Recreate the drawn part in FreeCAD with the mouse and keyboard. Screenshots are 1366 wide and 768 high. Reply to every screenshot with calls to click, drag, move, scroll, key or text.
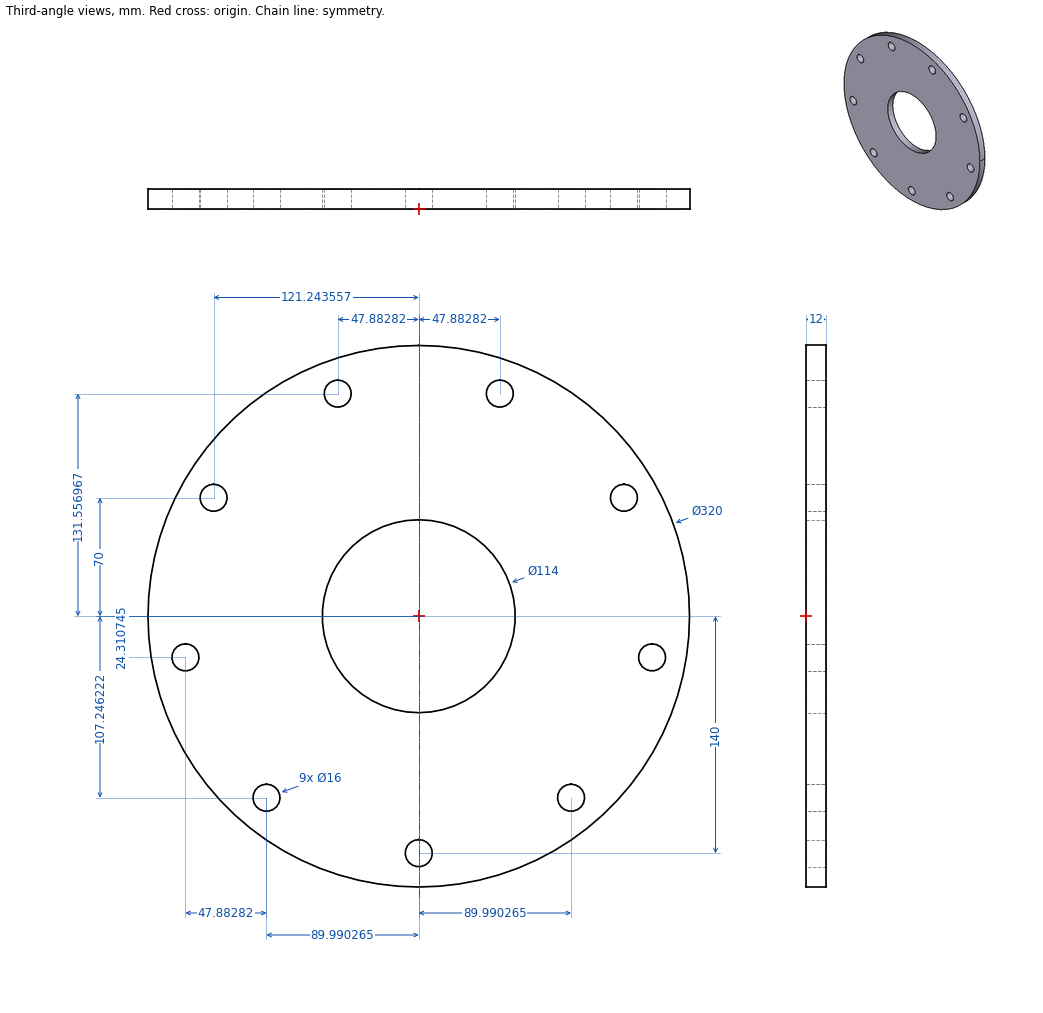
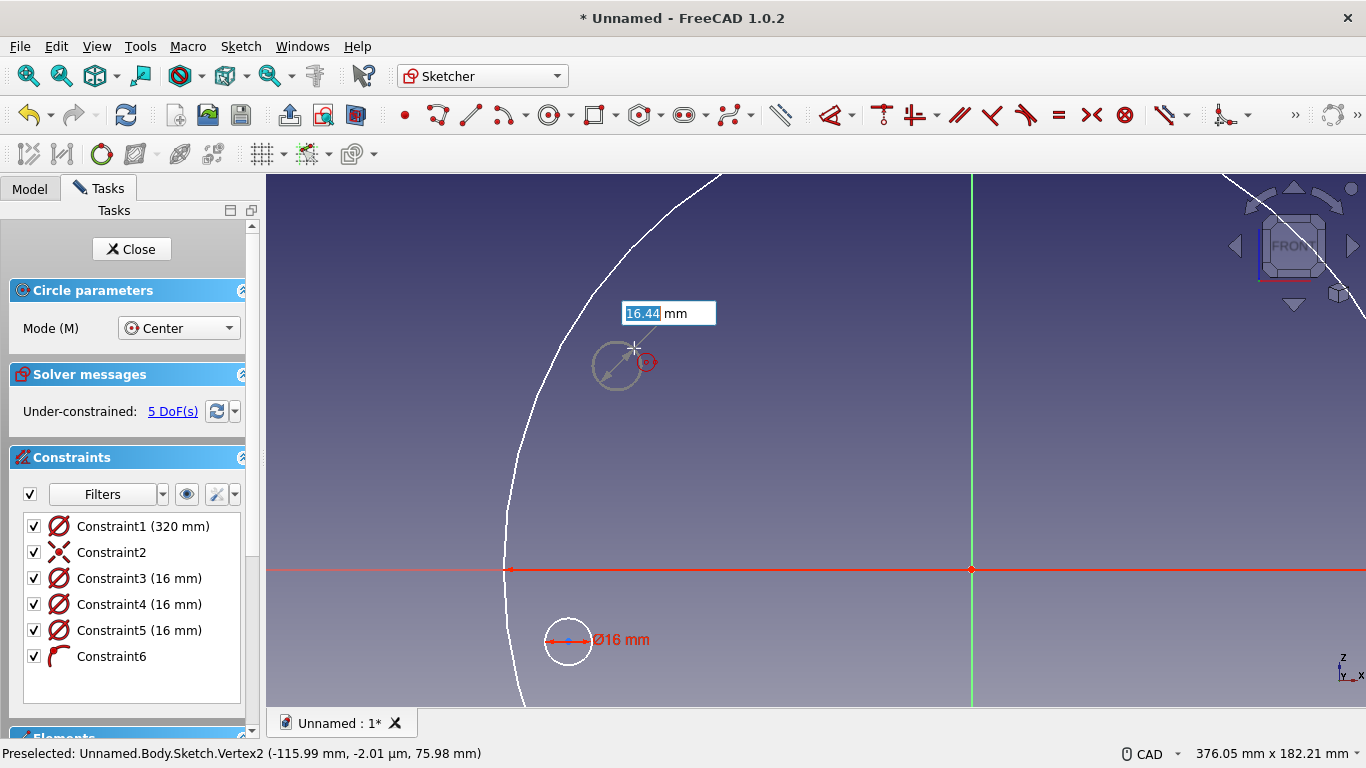
text(16)
key(Return)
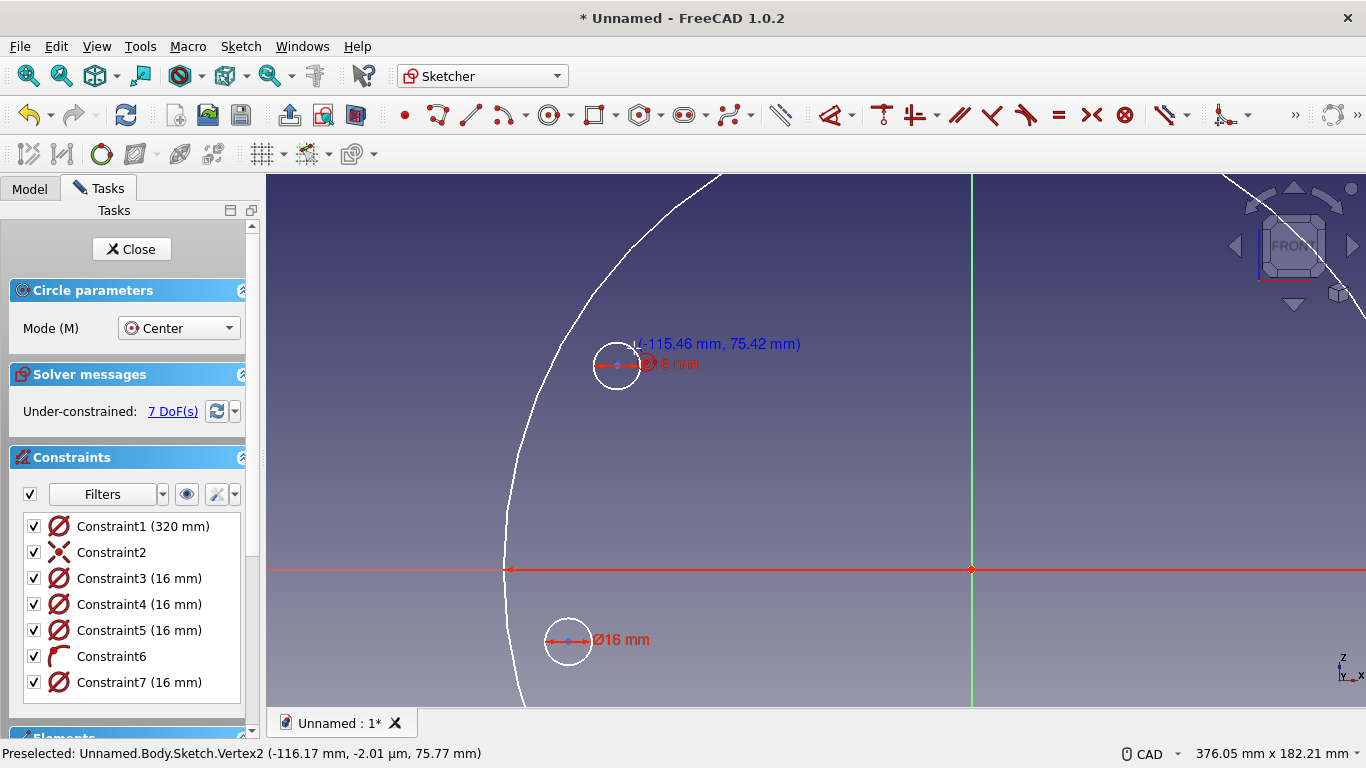
click(972, 570)
move(1090, 452)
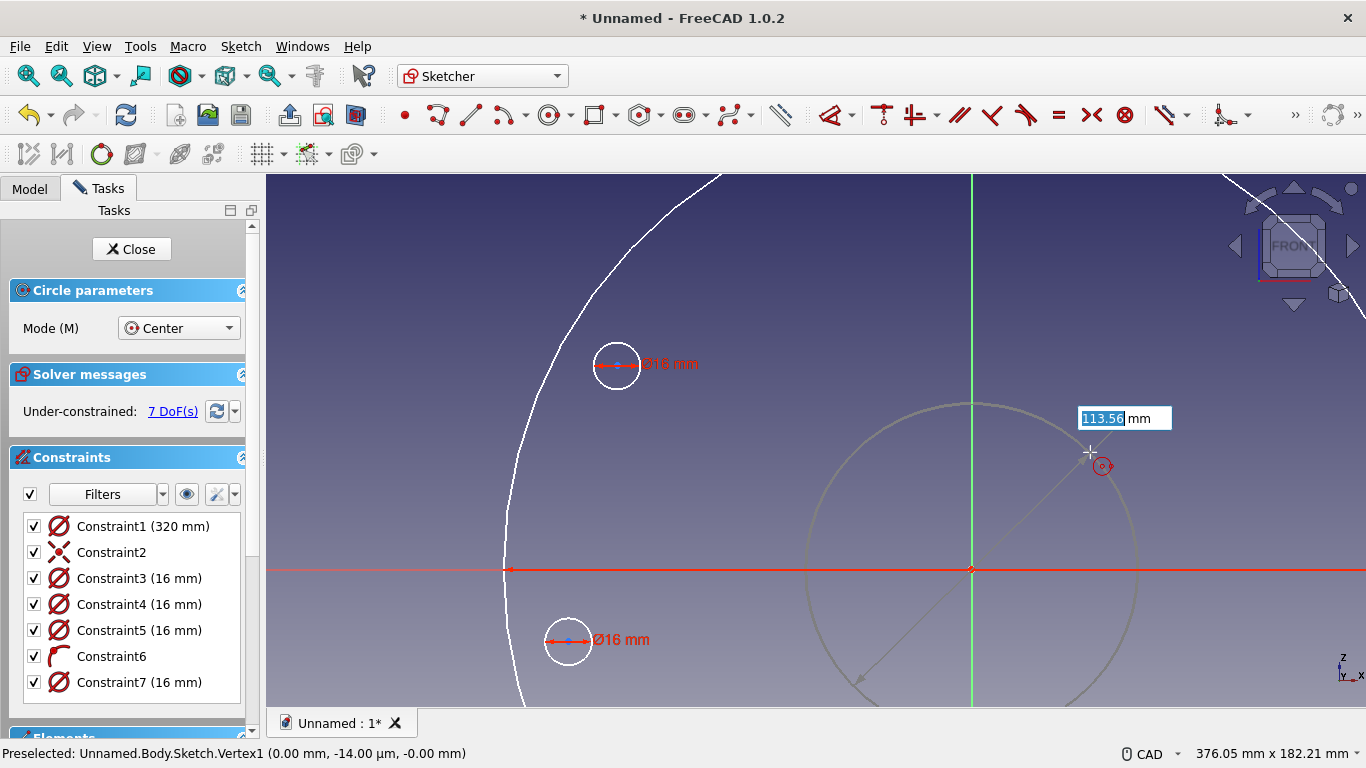
text(114)
key(Return)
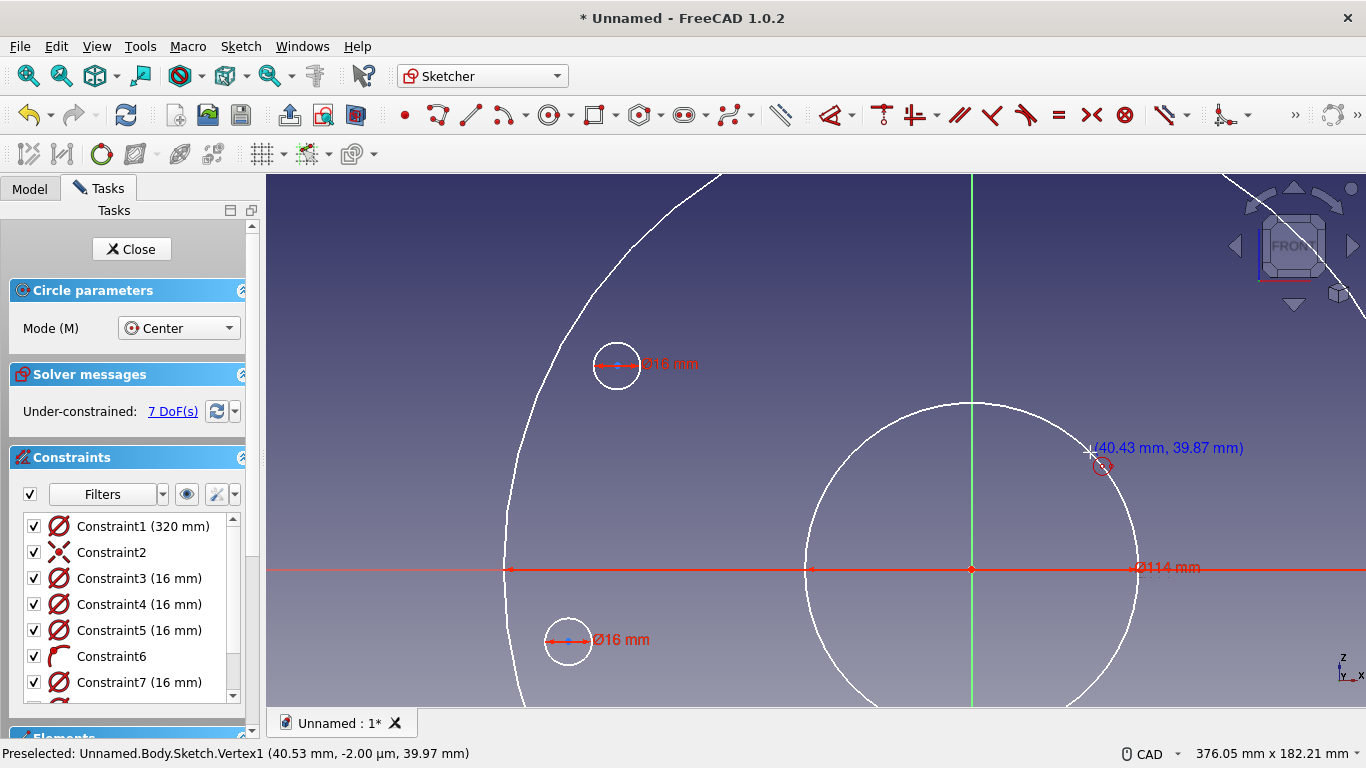
scroll(617, 365, down, 5)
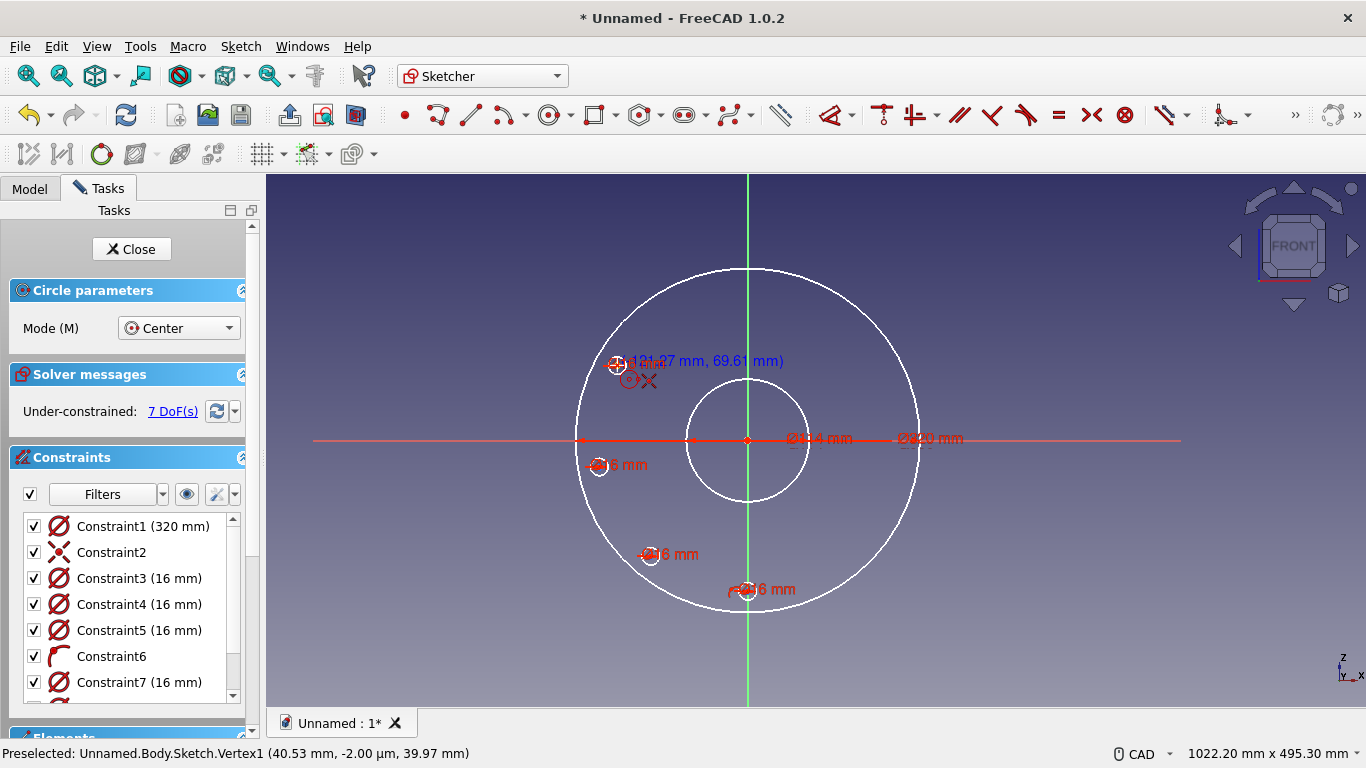
scroll(696, 299, up, 5)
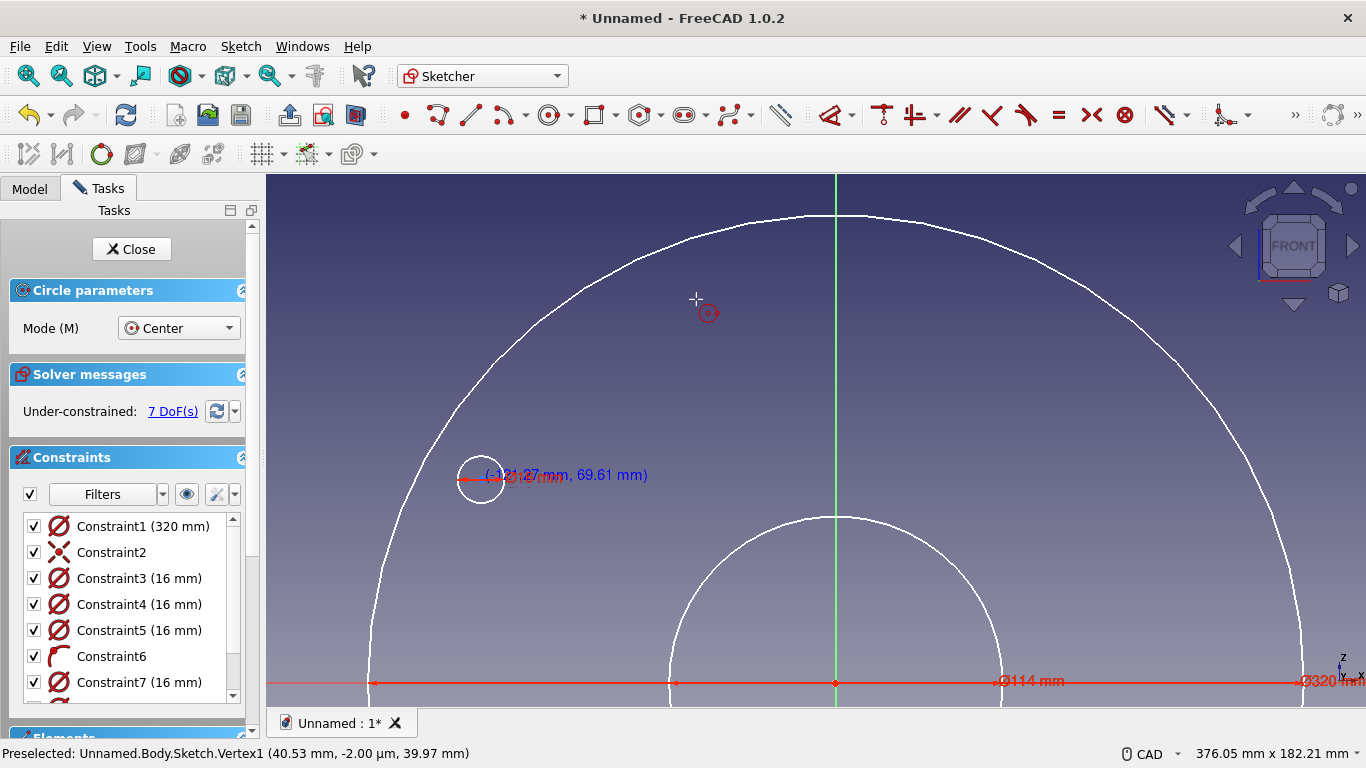
click(696, 298)
move(712, 282)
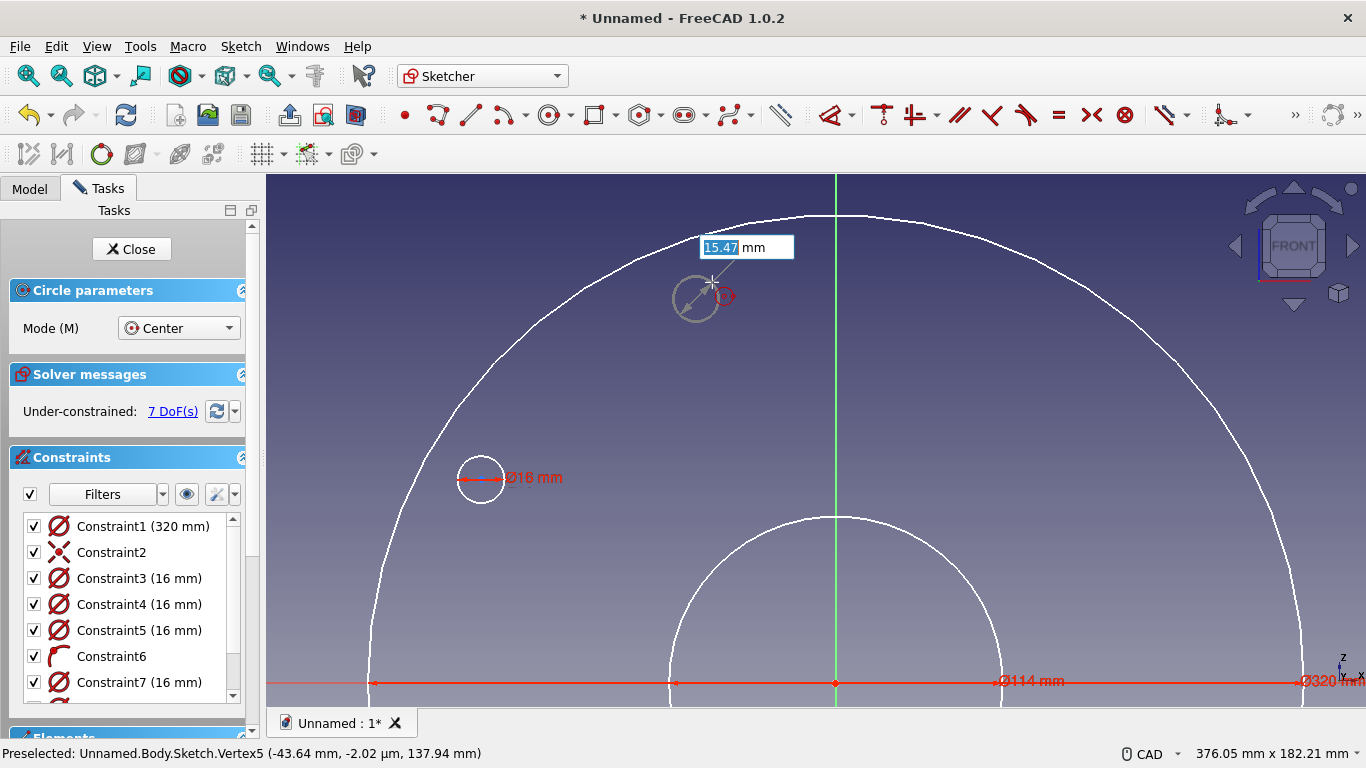
text(16)
key(Return)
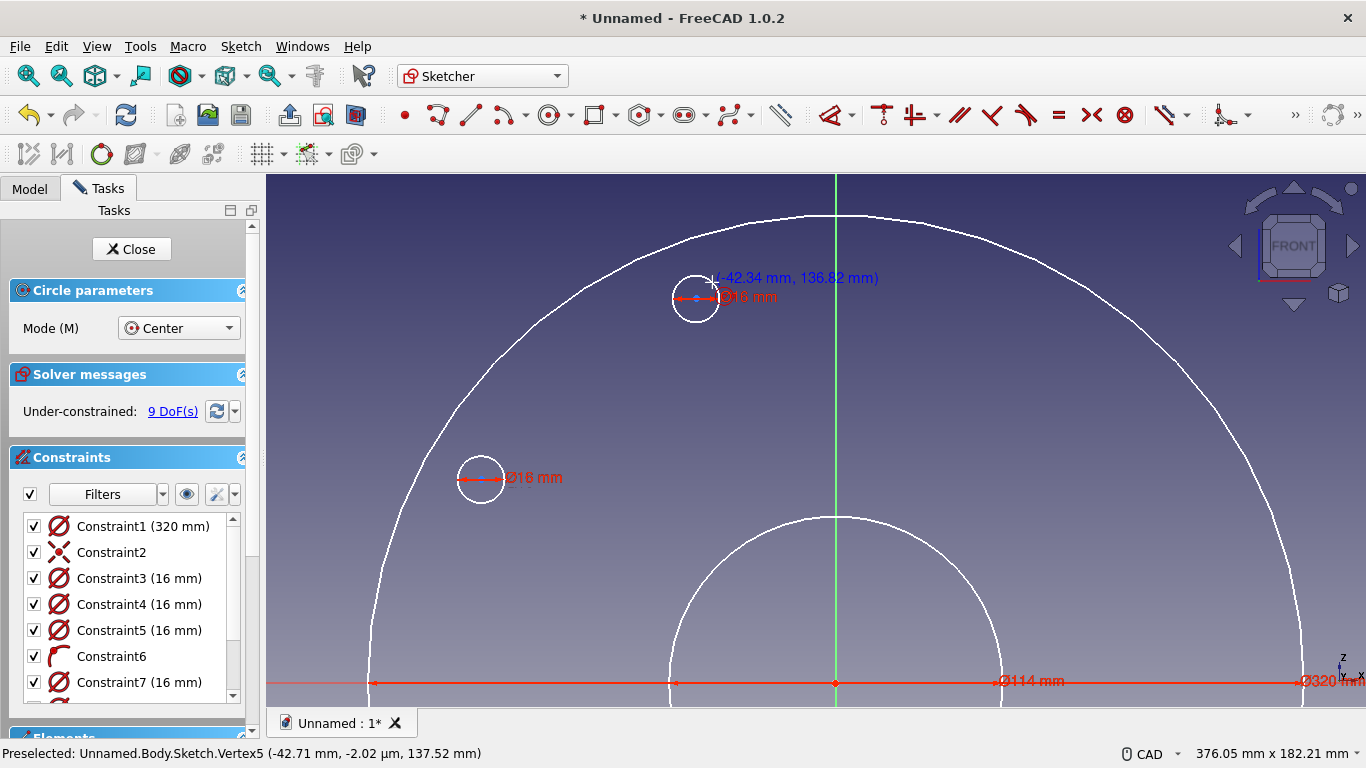
scroll(696, 299, down, 5)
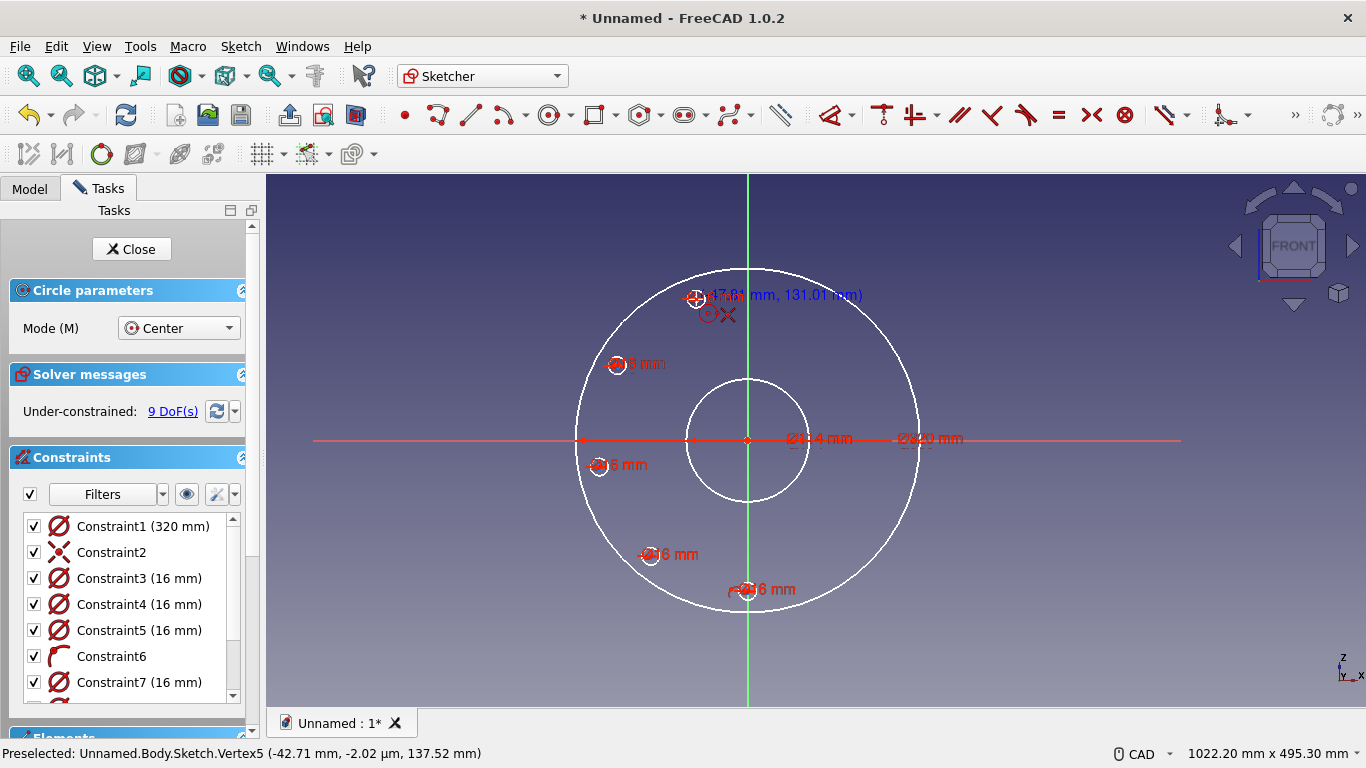
scroll(845, 556, up, 5)